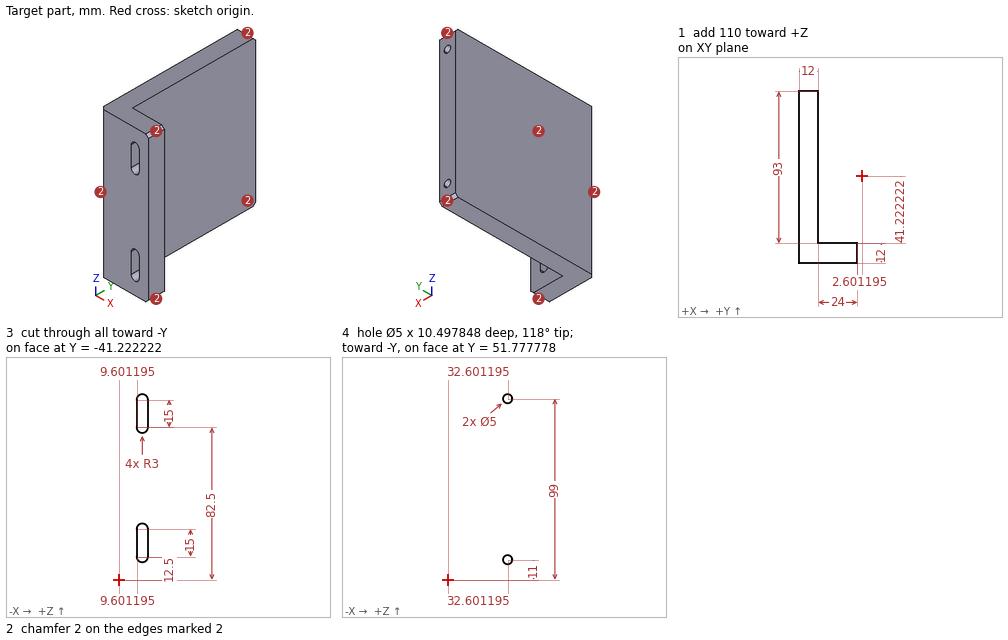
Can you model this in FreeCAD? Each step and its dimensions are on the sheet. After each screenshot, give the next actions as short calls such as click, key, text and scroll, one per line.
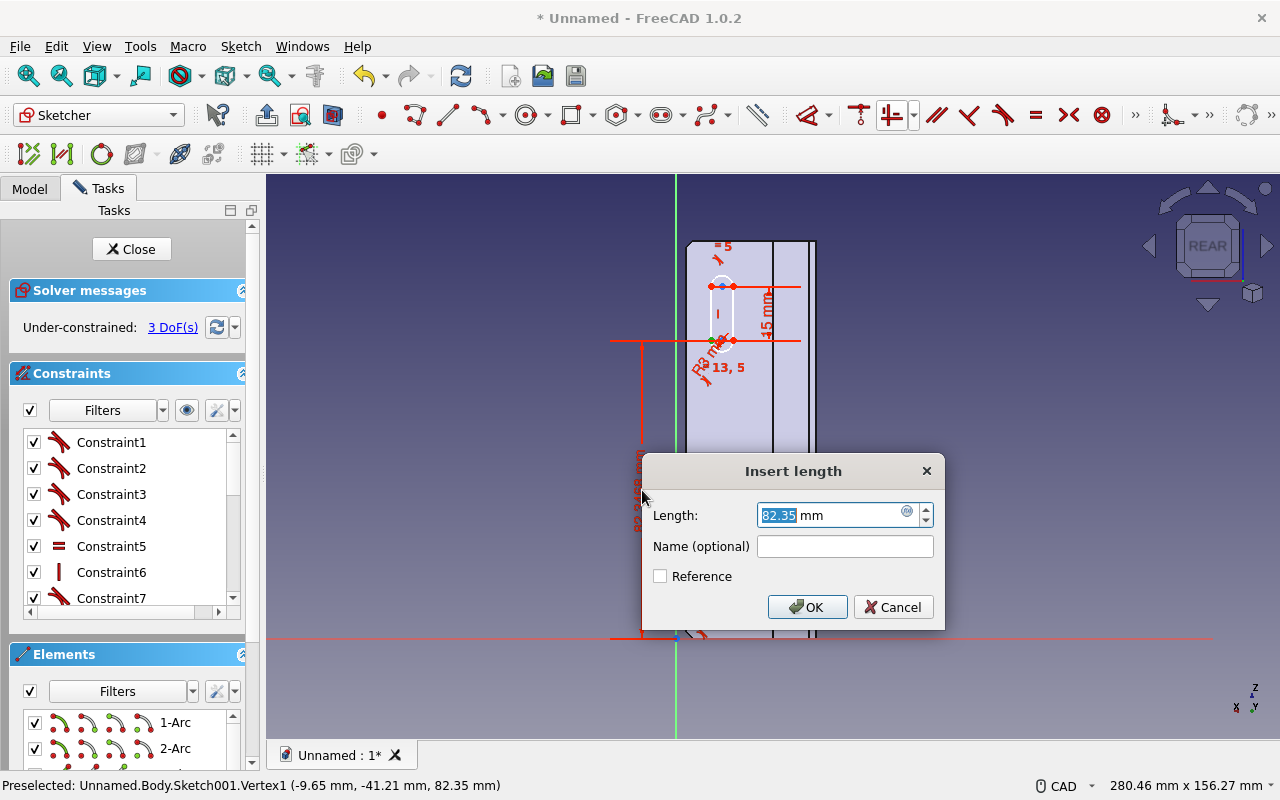
text(82.5)
key(Return)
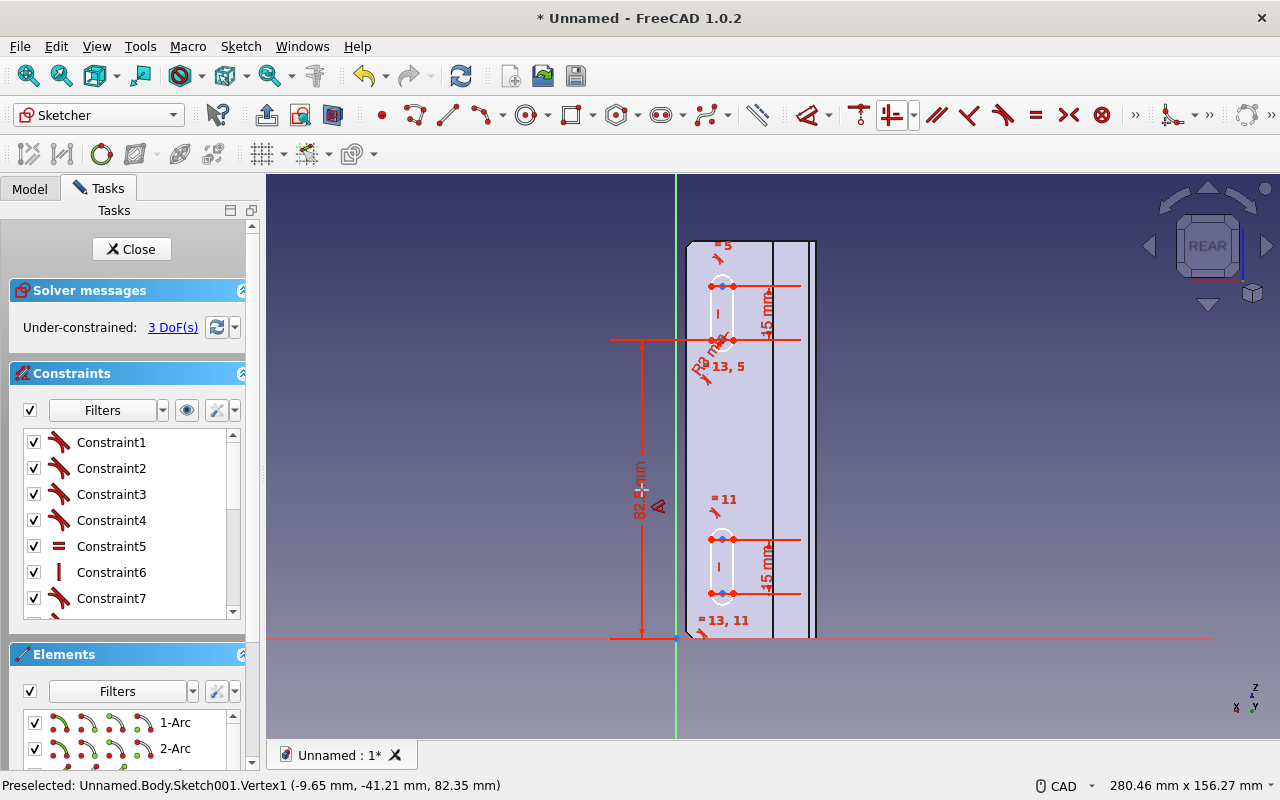
click(711, 594)
click(642, 616)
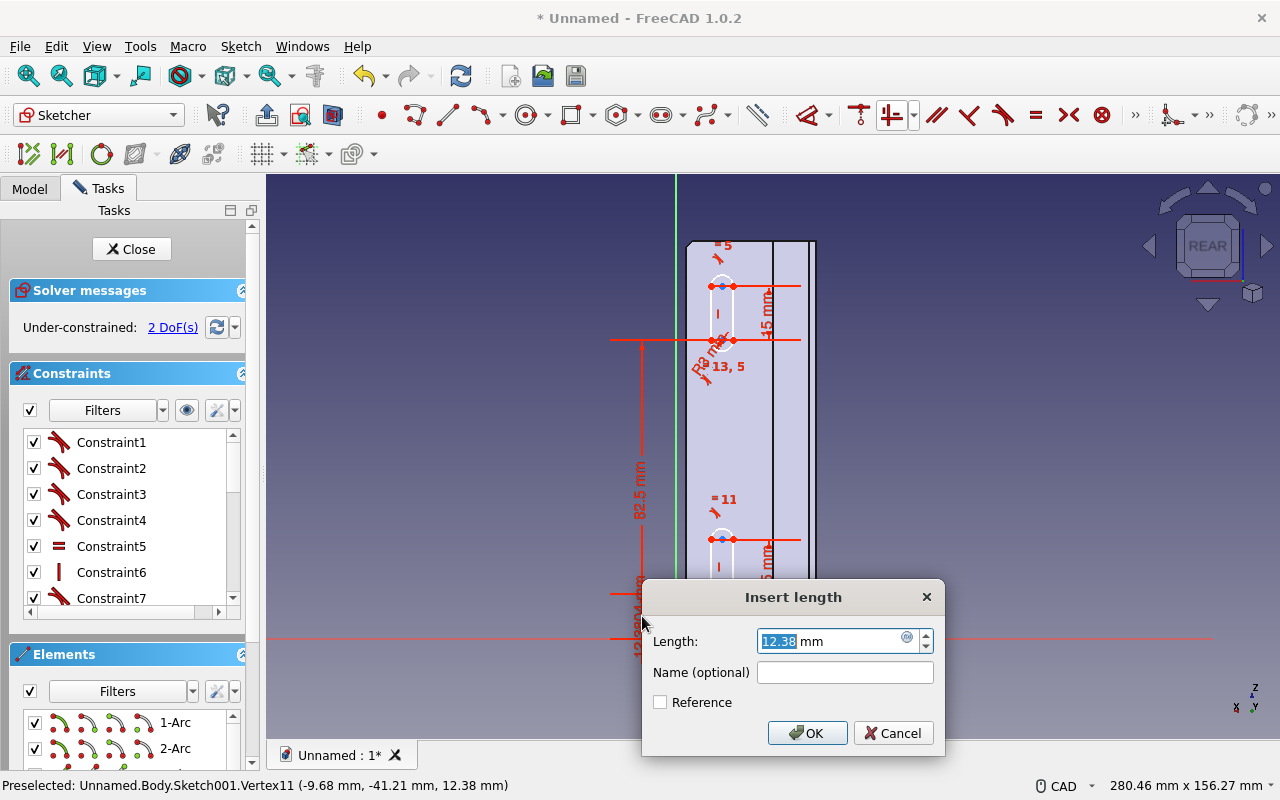
text(12.5)
key(Return)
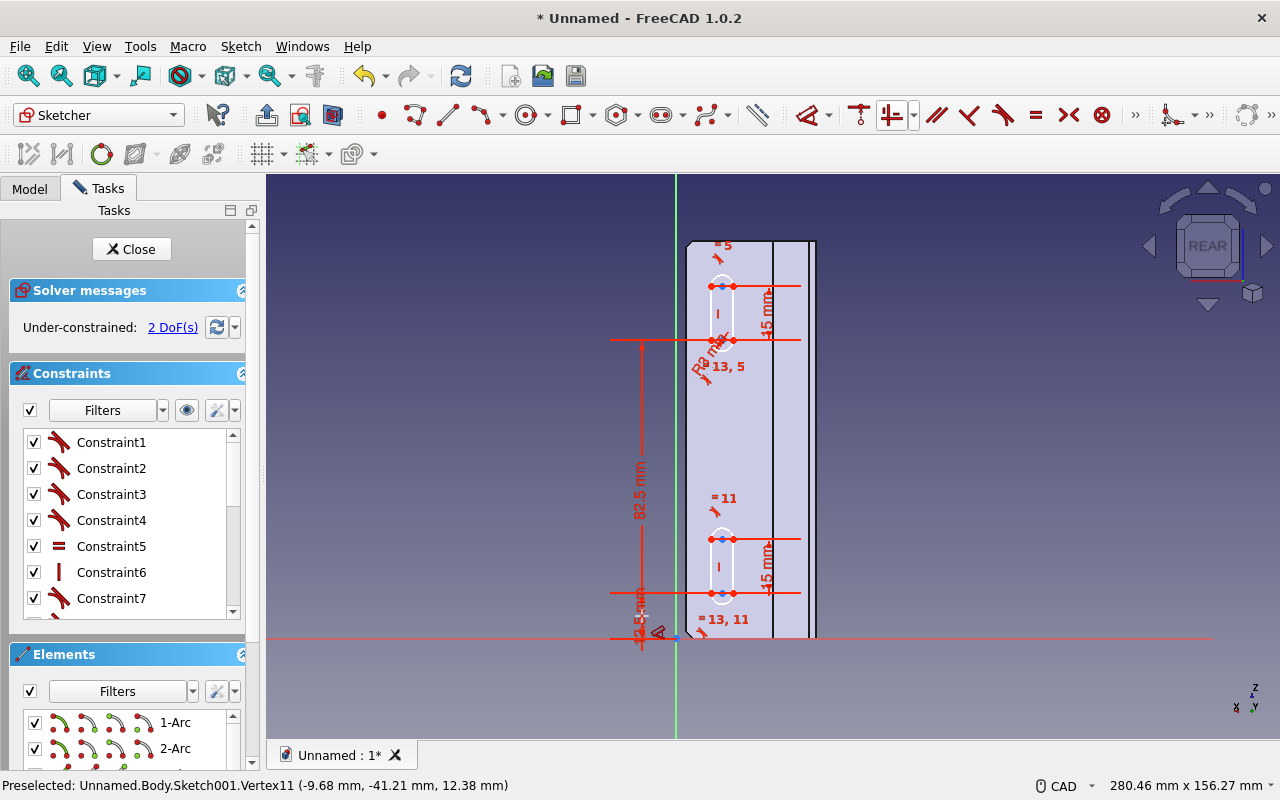
click(711, 340)
click(694, 673)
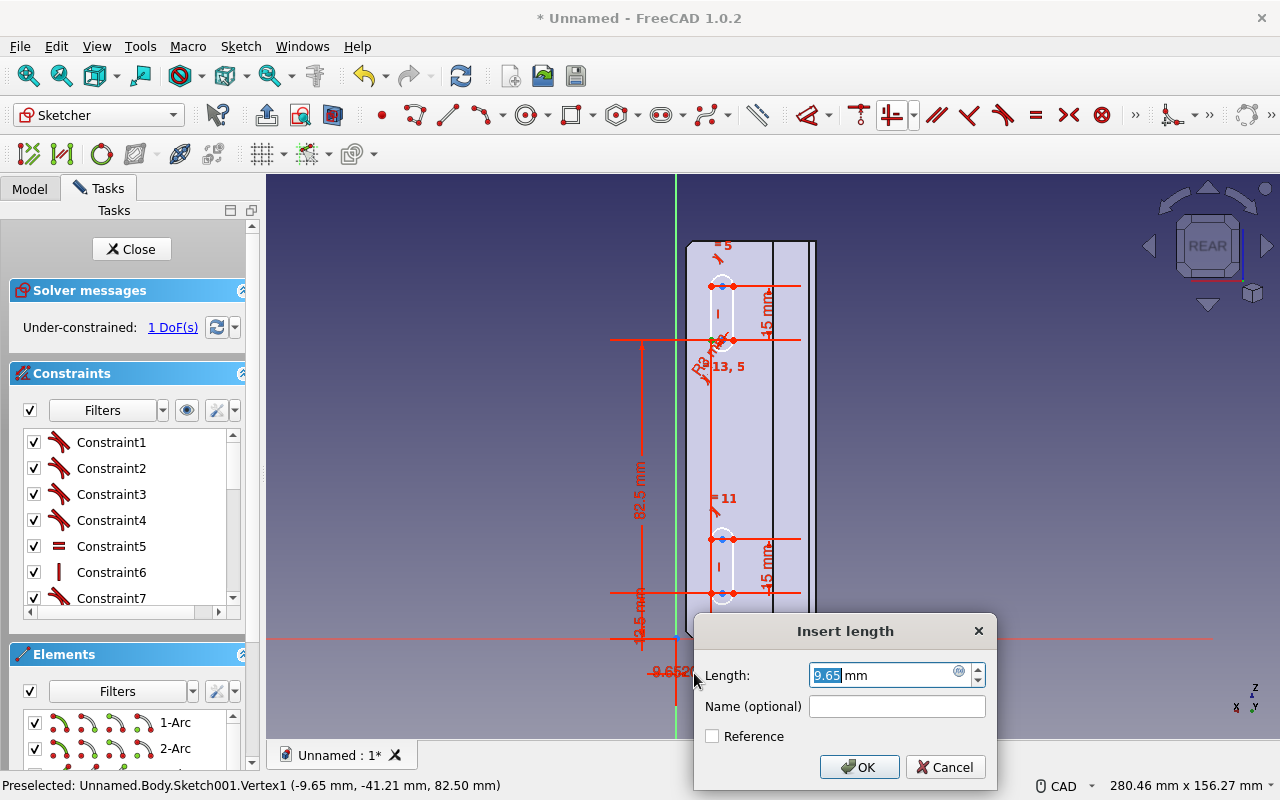
text(9.601195)
key(Return)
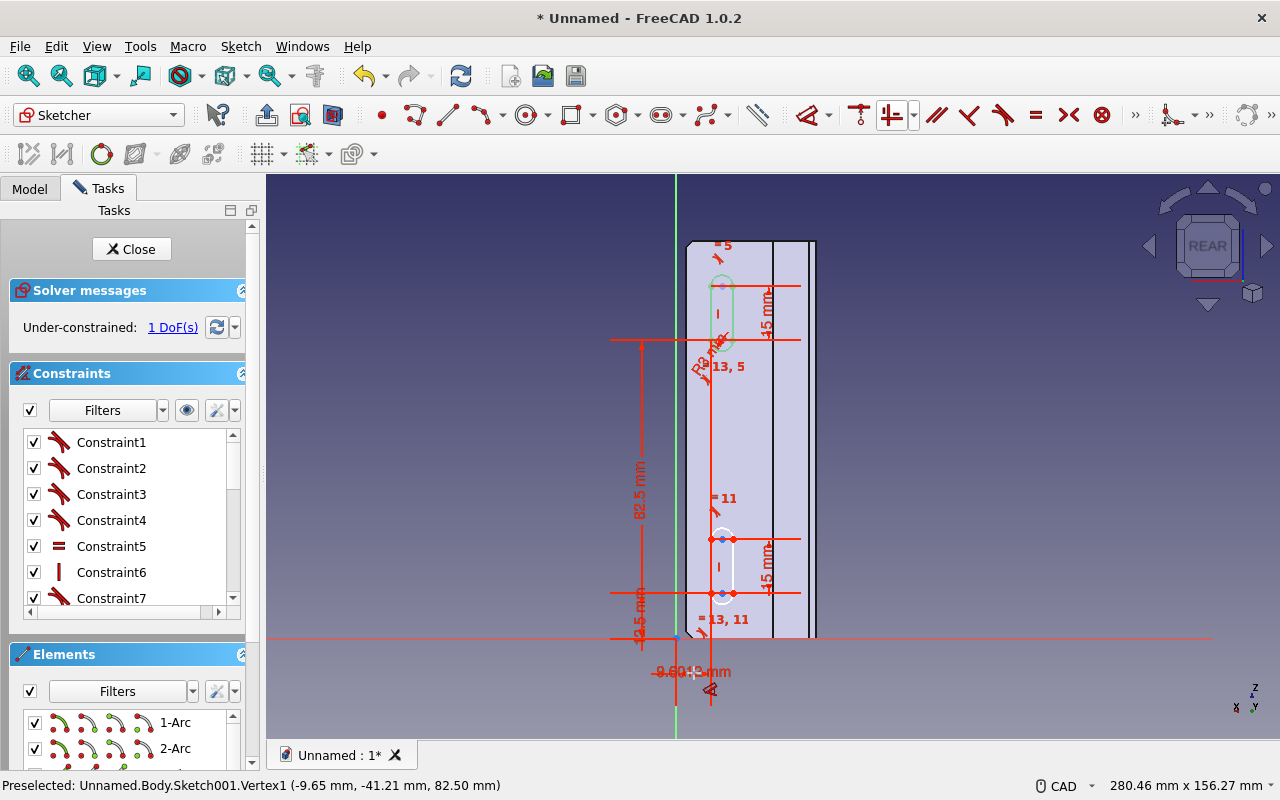
click(711, 593)
click(694, 559)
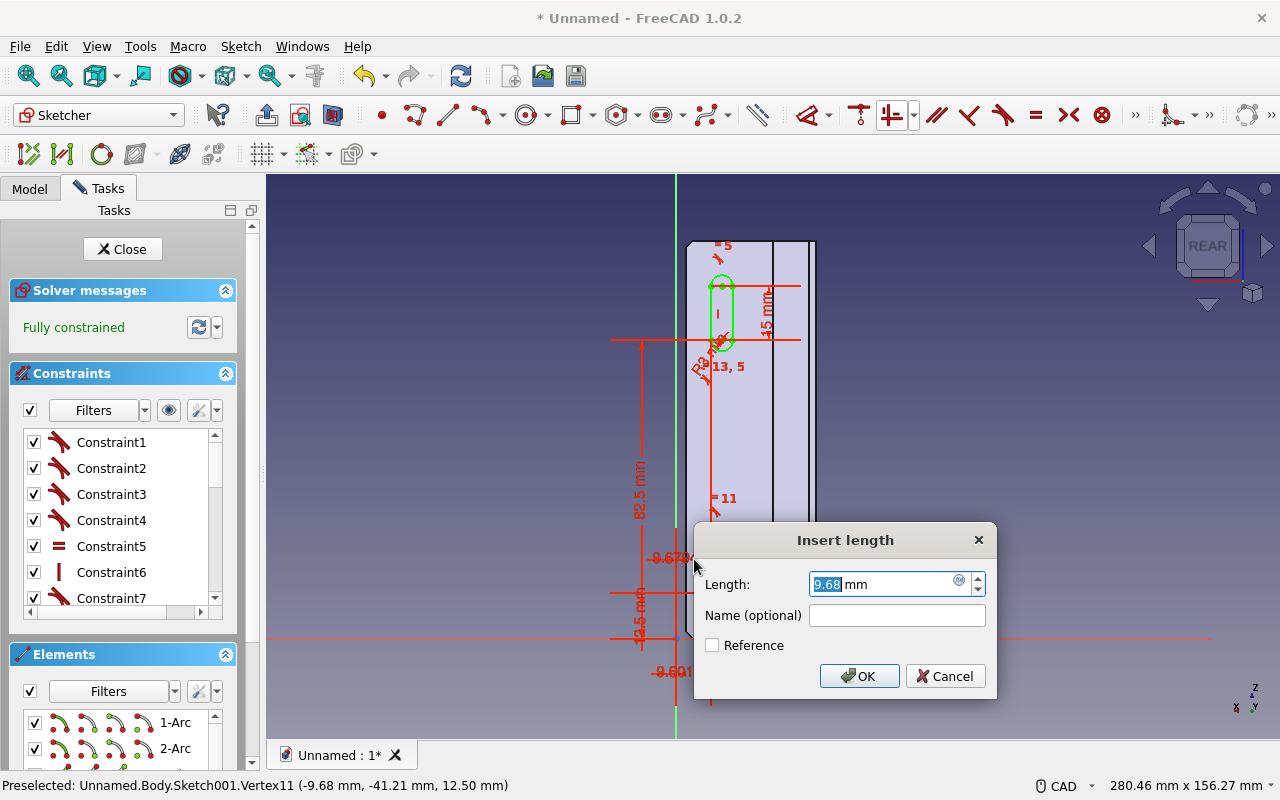
text(9.601195)
key(Return)
key(Escape)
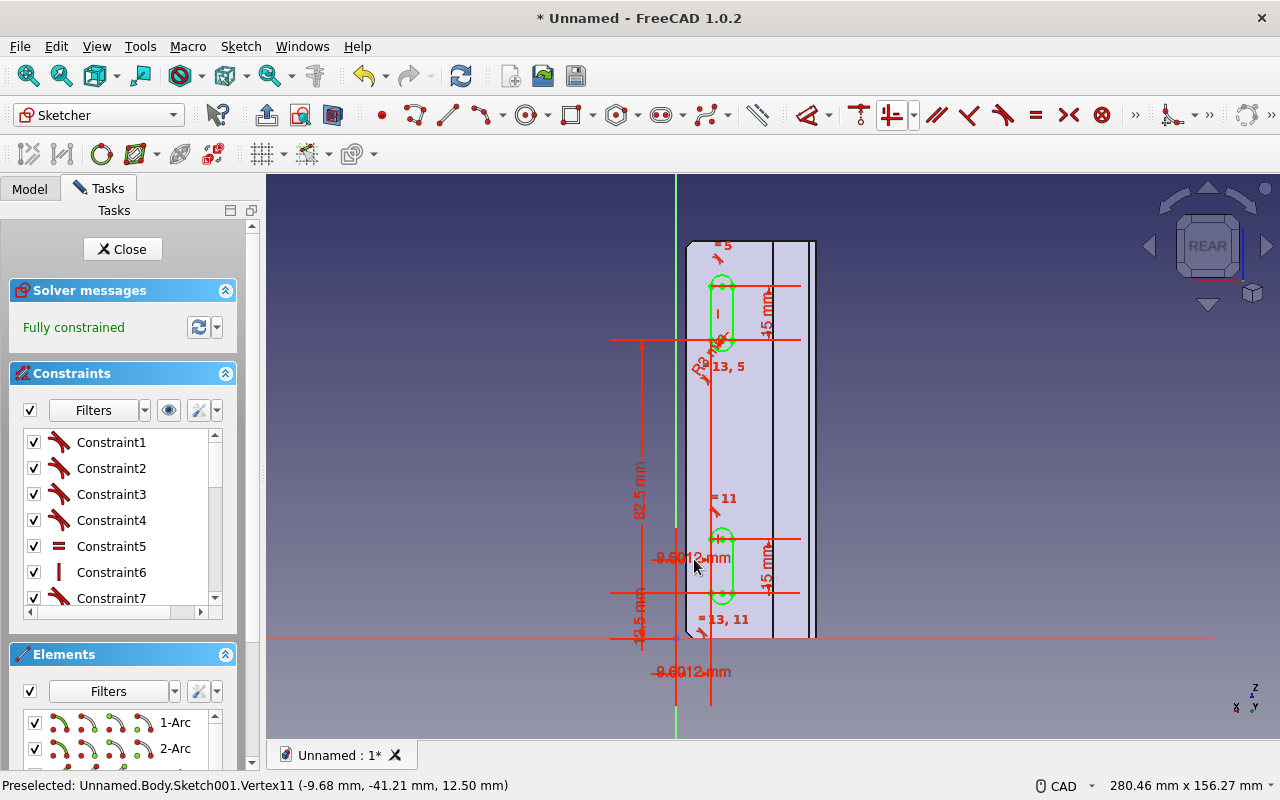
click(123, 249)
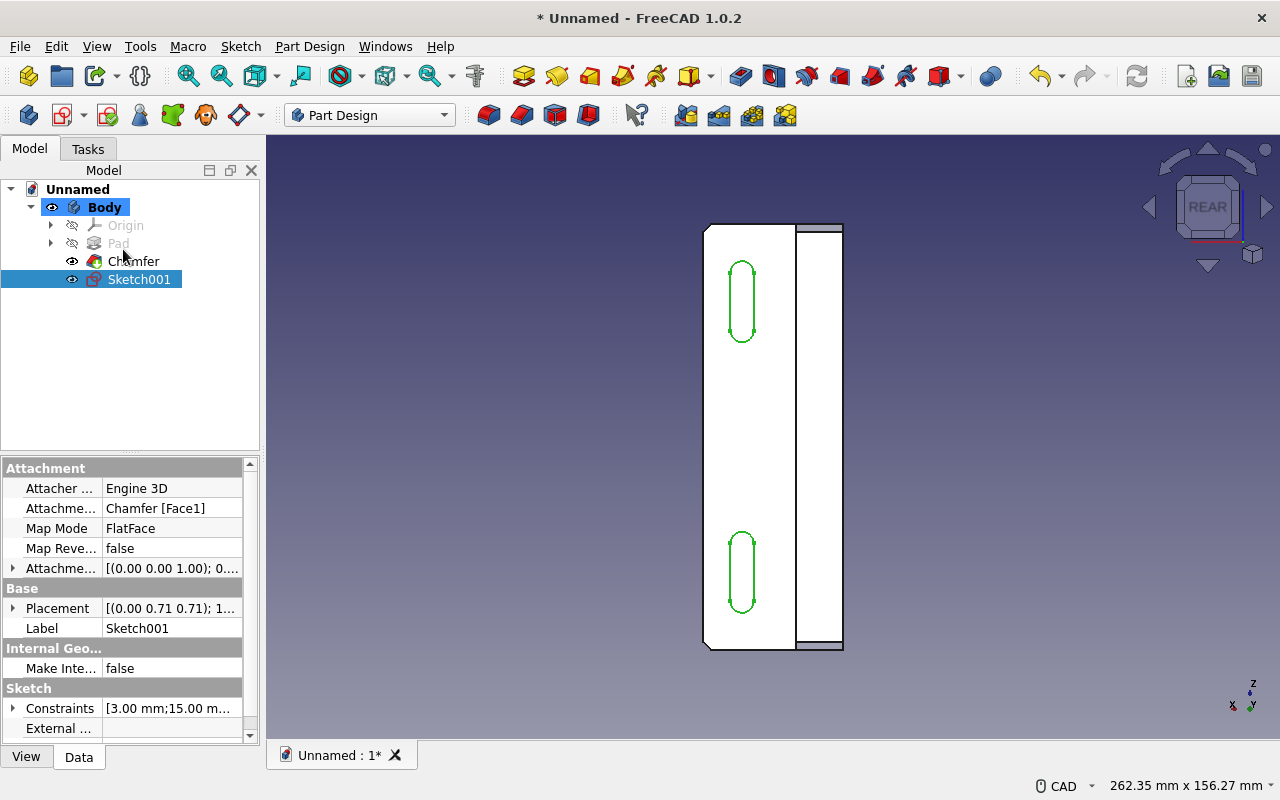
click(741, 76)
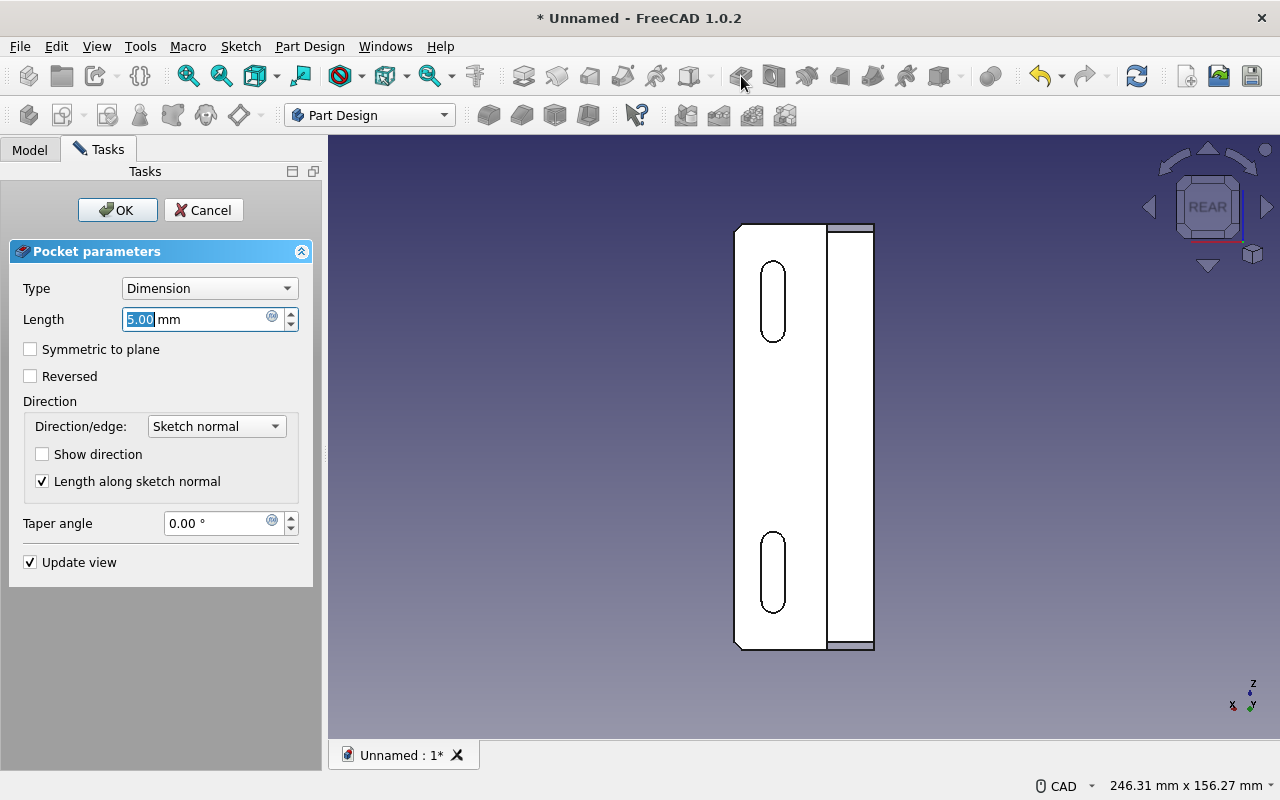
click(210, 288)